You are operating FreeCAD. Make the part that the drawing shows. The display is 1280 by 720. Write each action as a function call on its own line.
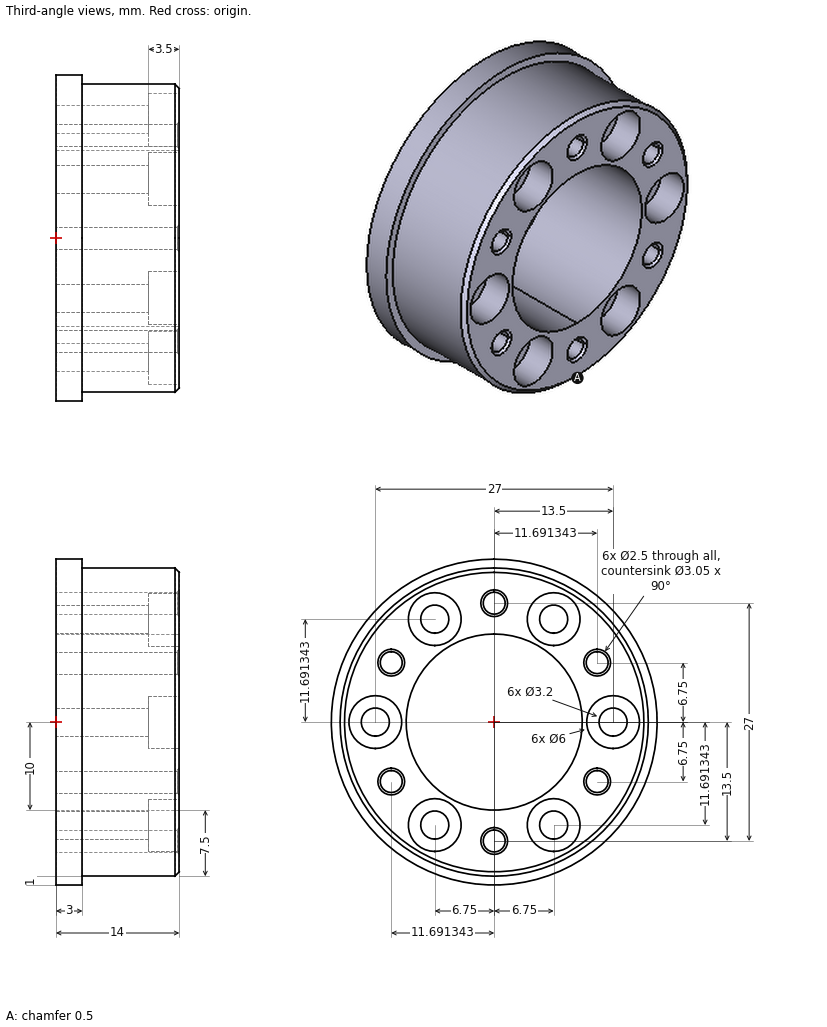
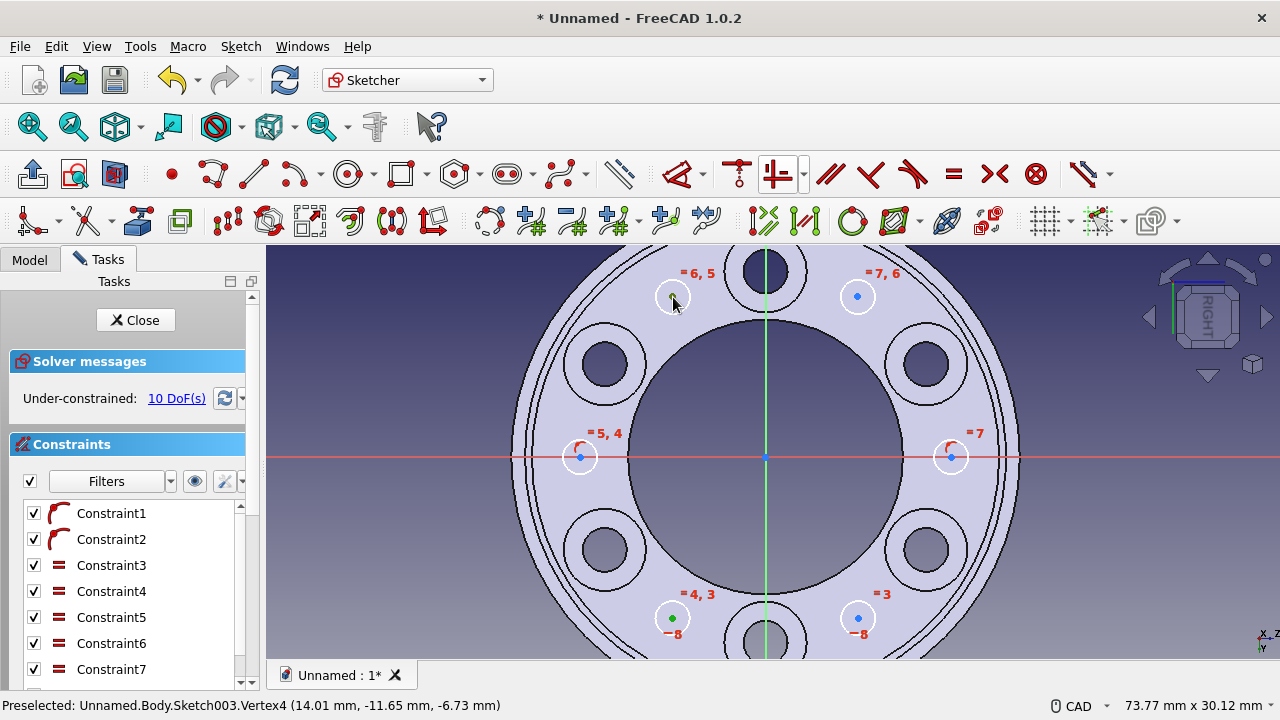
click(804, 174)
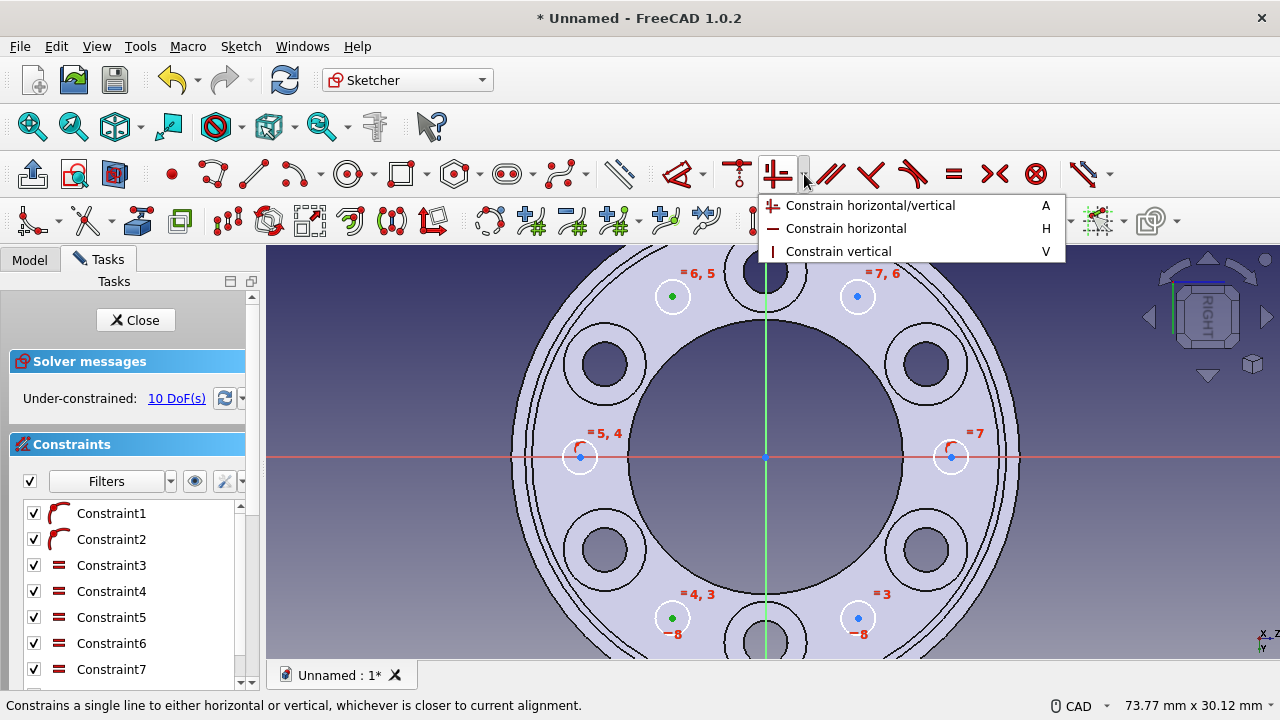
click(912, 252)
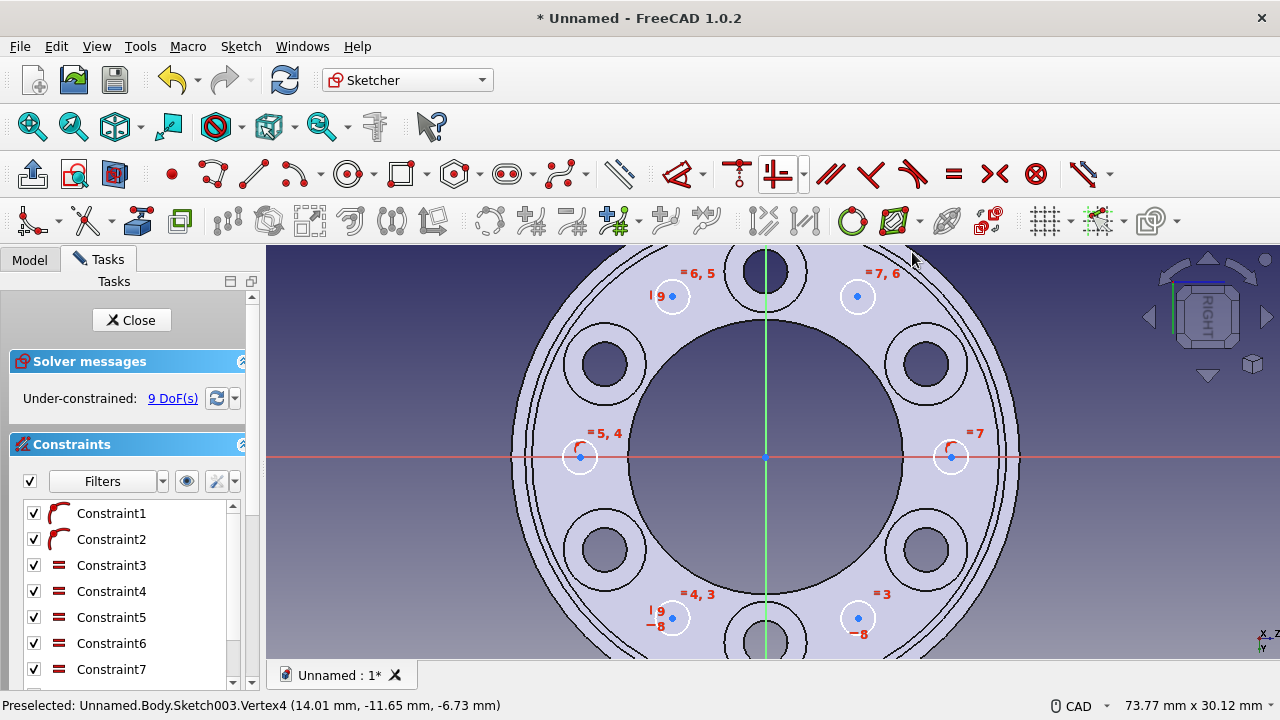
click(858, 618)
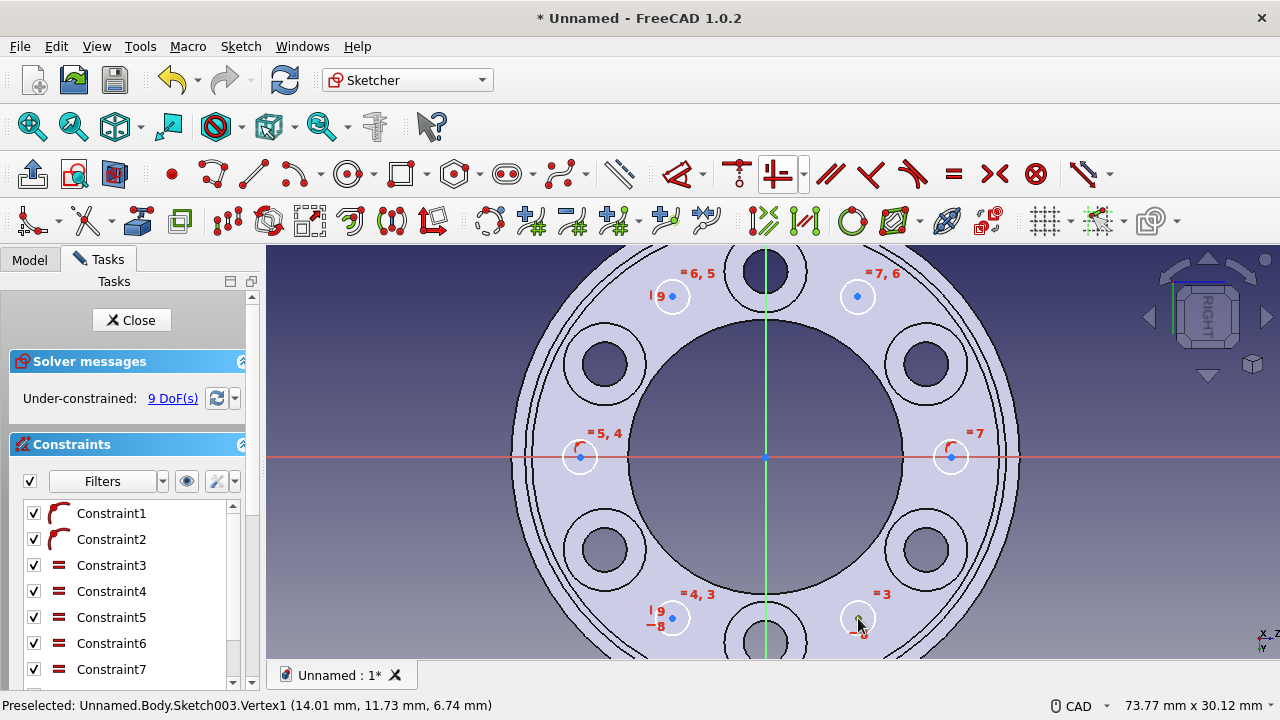
click(858, 297)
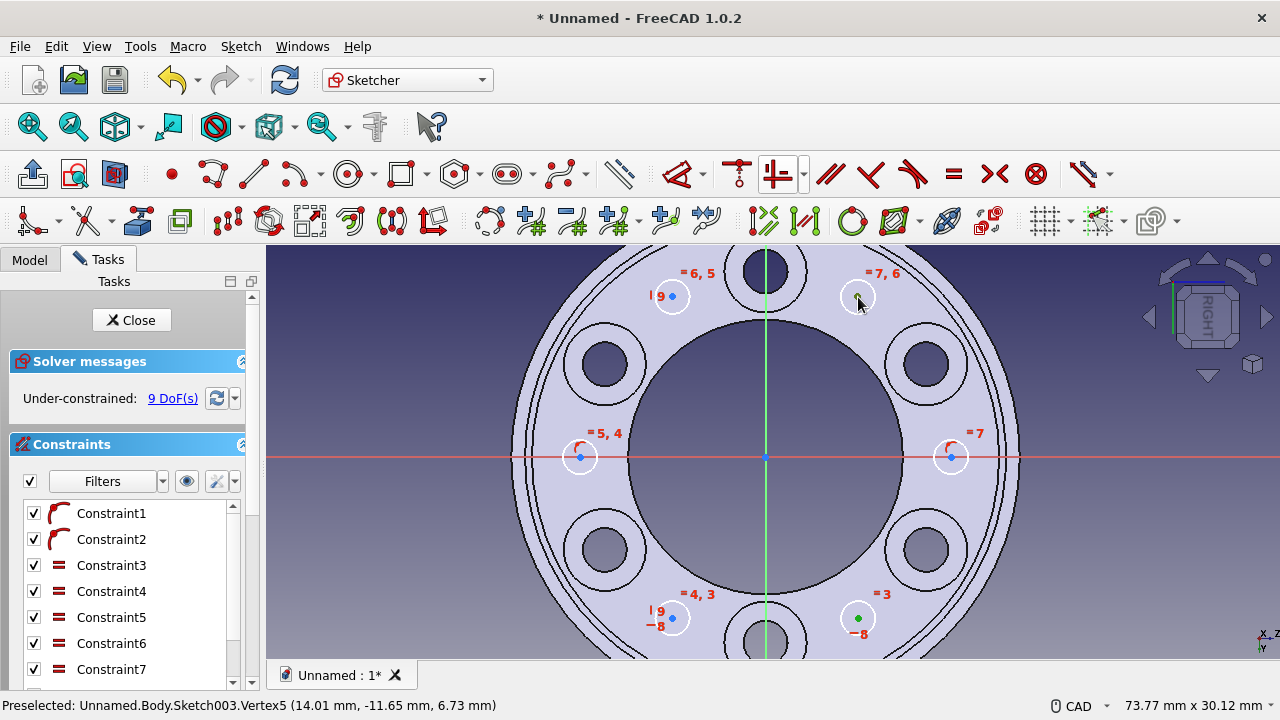
key(v)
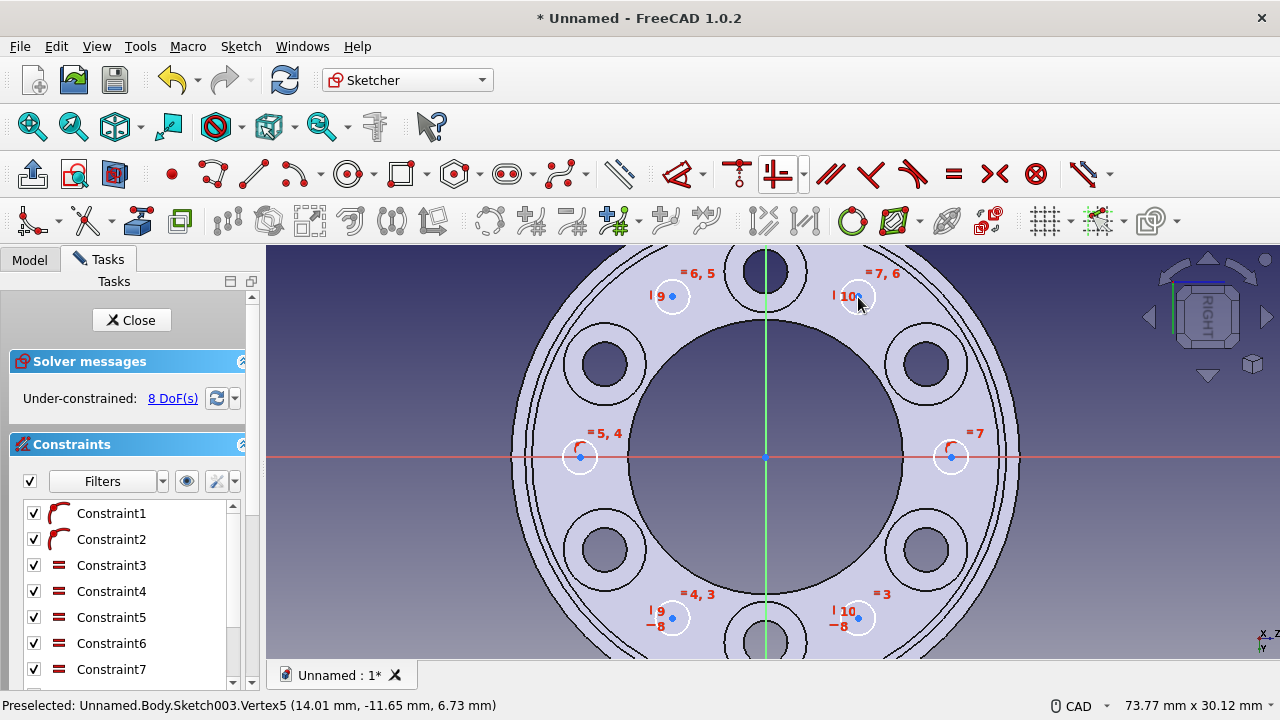
click(673, 297)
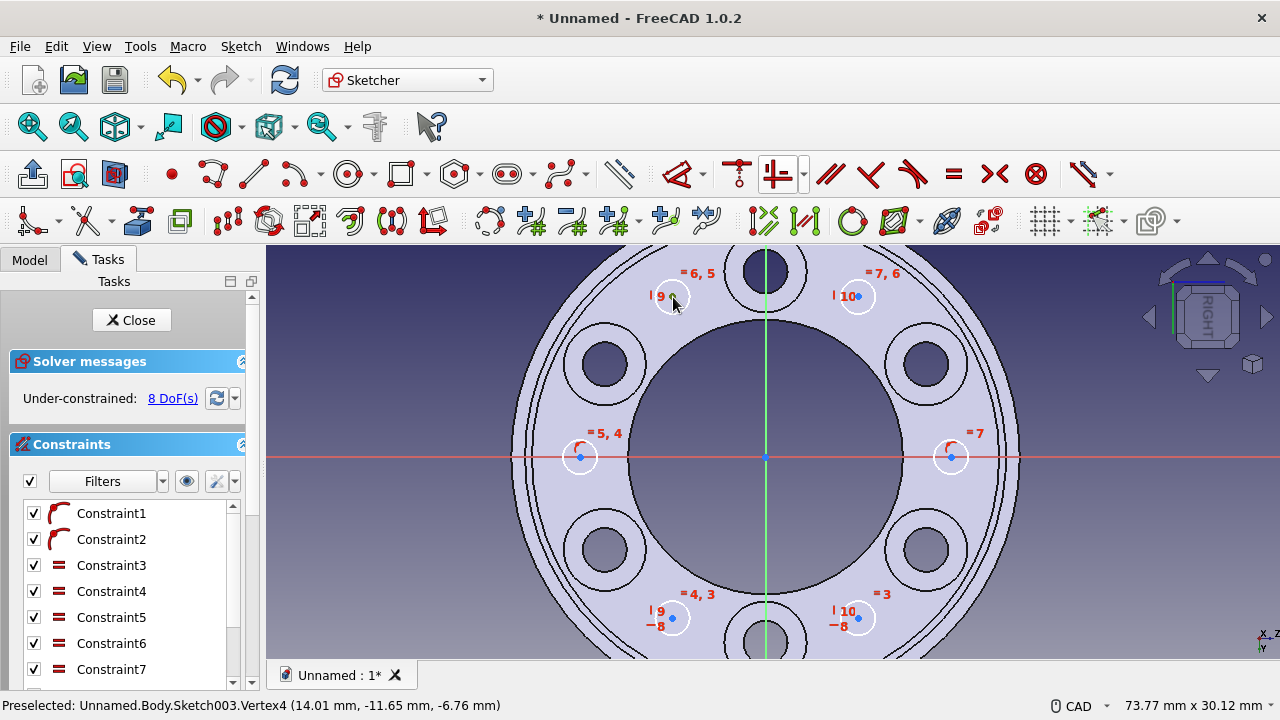
click(858, 297)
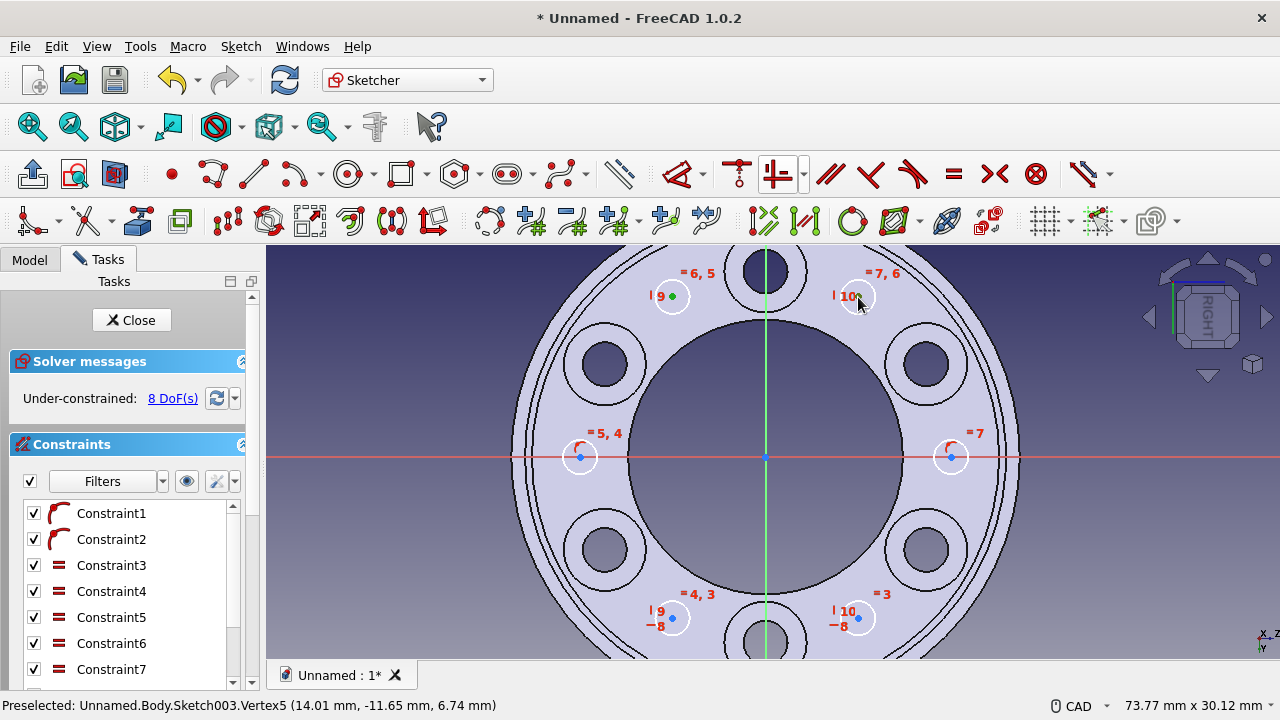
click(804, 174)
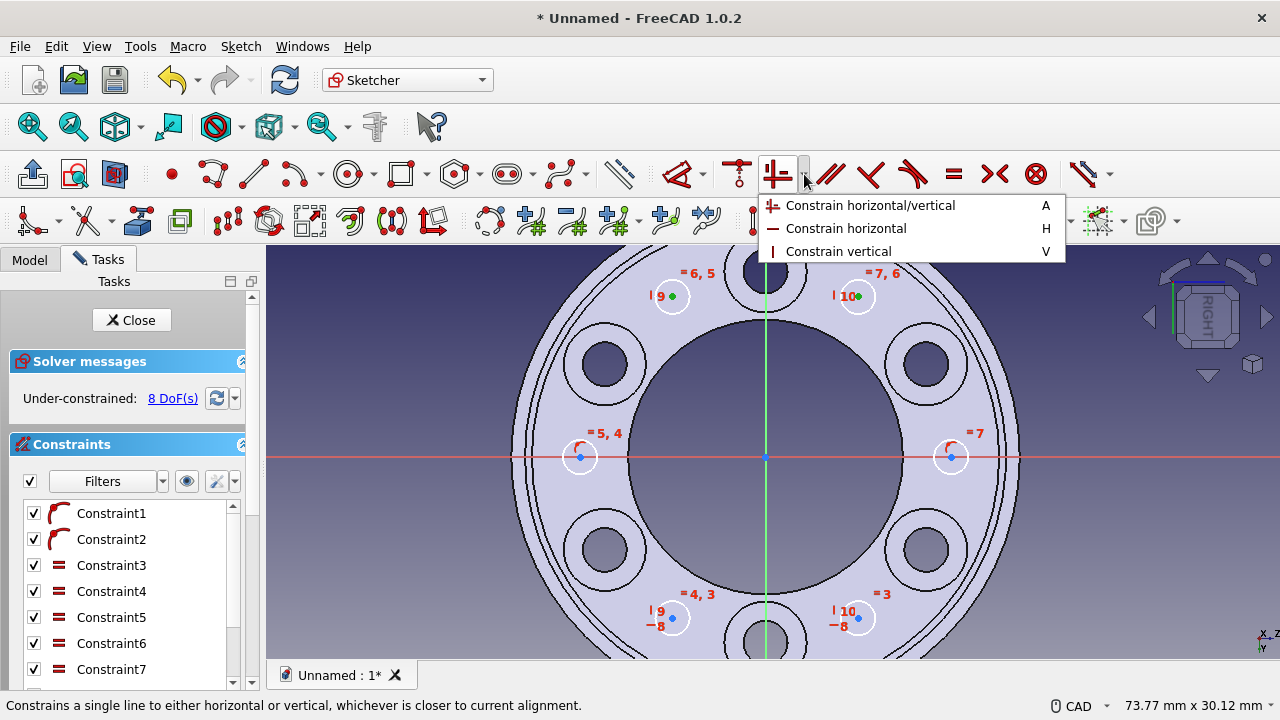
click(912, 228)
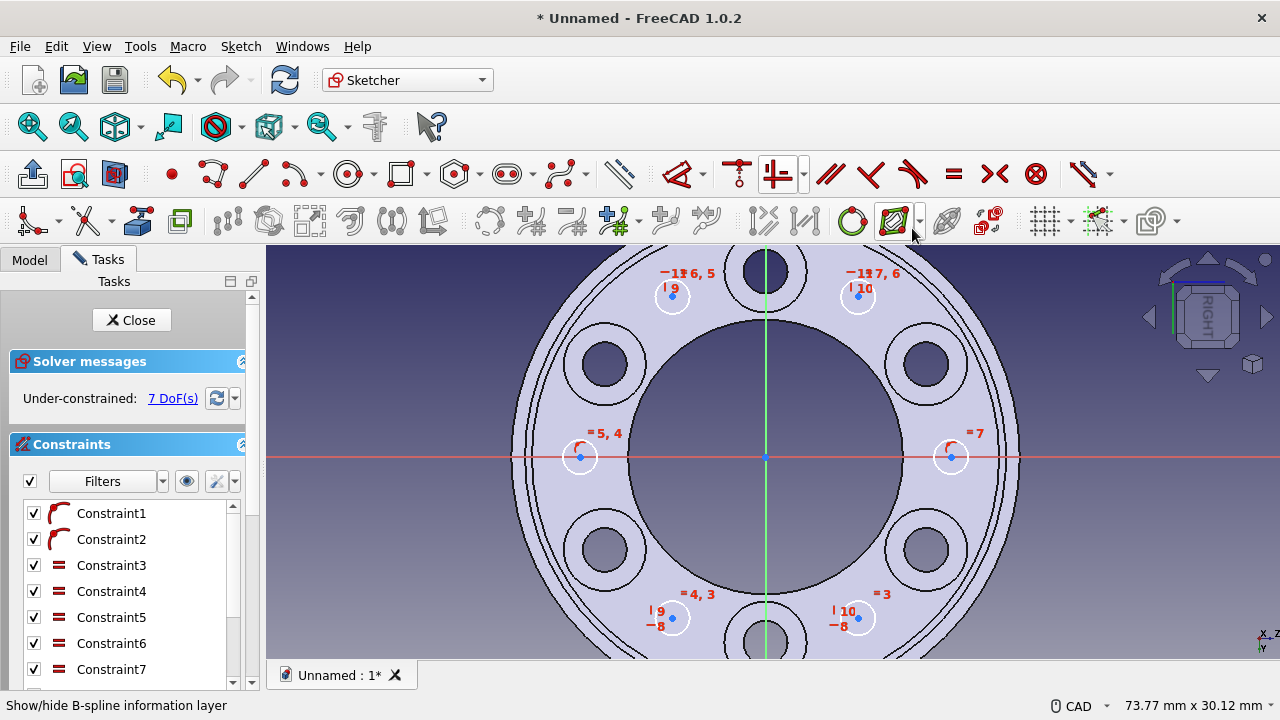
click(676, 174)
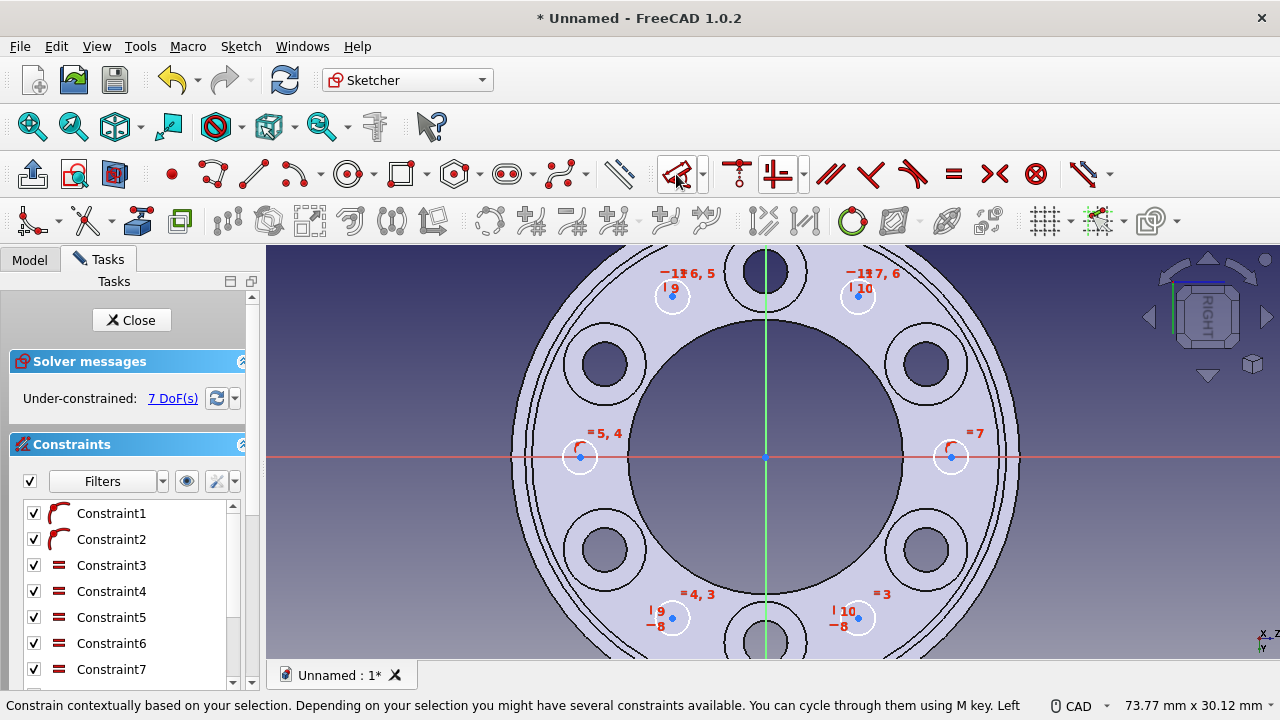
click(870, 606)
click(892, 583)